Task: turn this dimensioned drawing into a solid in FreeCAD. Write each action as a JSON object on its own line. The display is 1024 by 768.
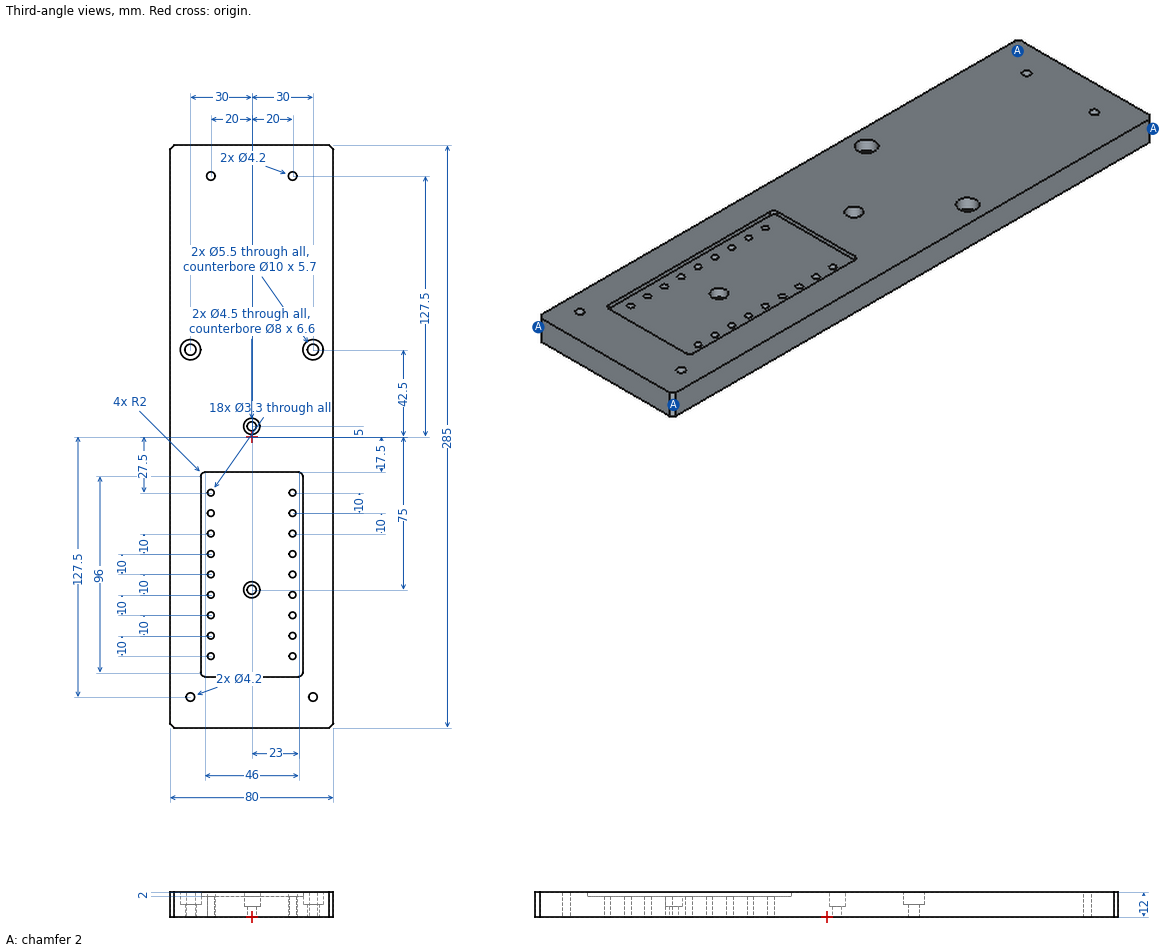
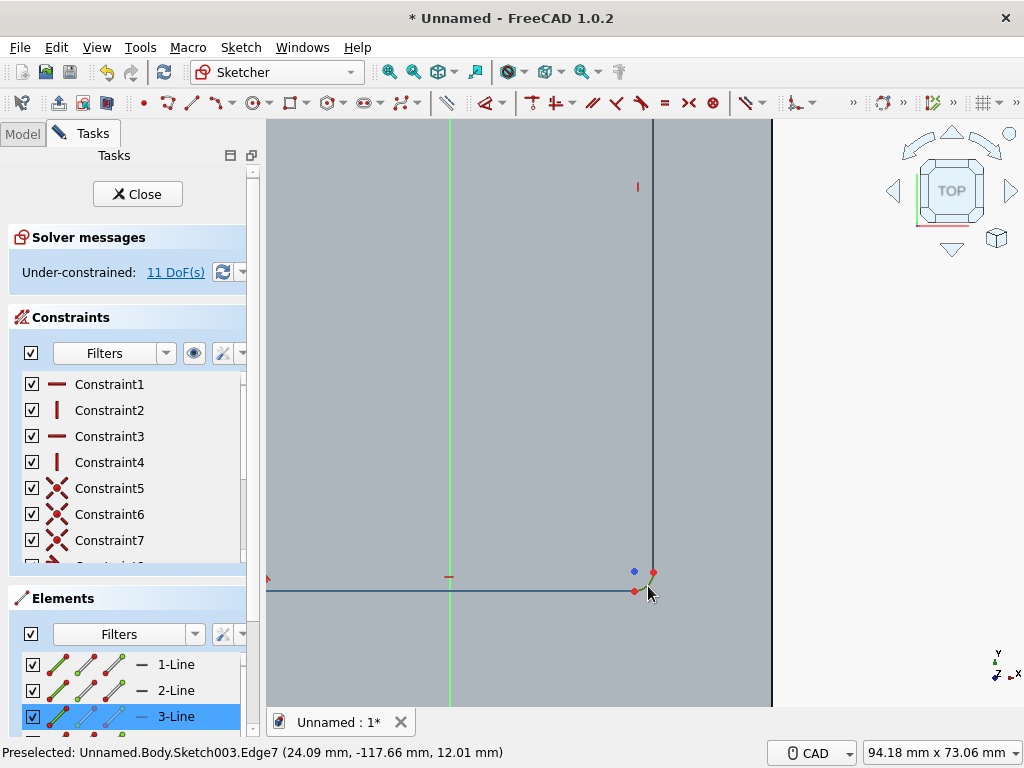
{"action": "key", "text": "t"}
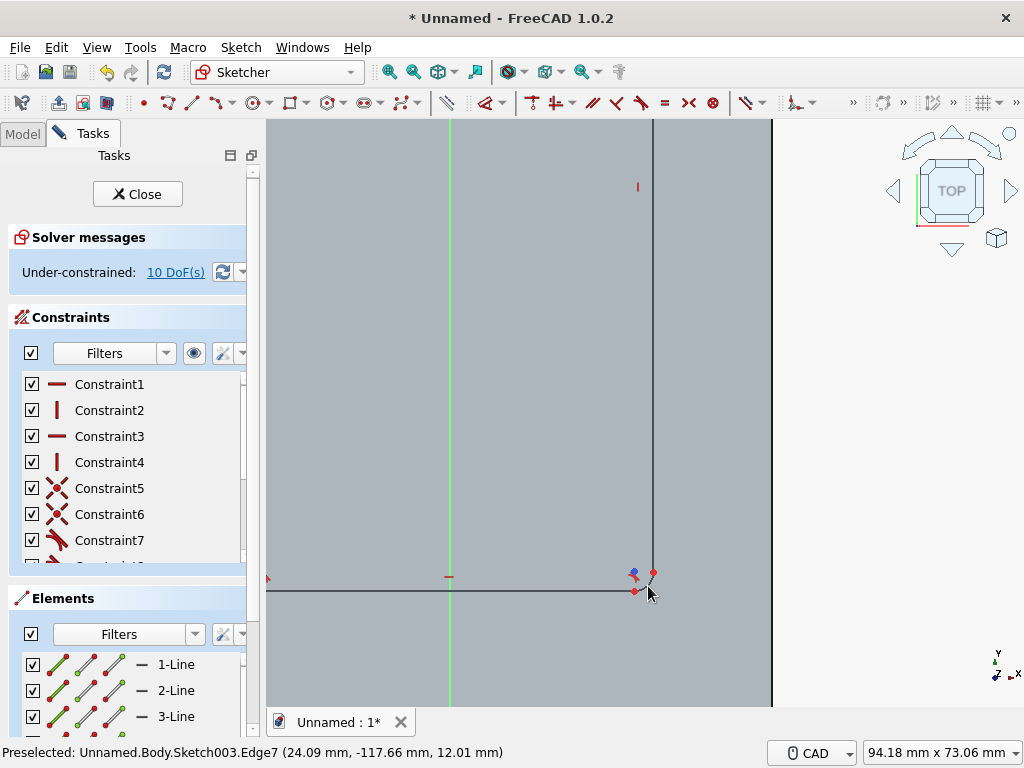
{"action": "left_click", "coordinate": [653, 341]}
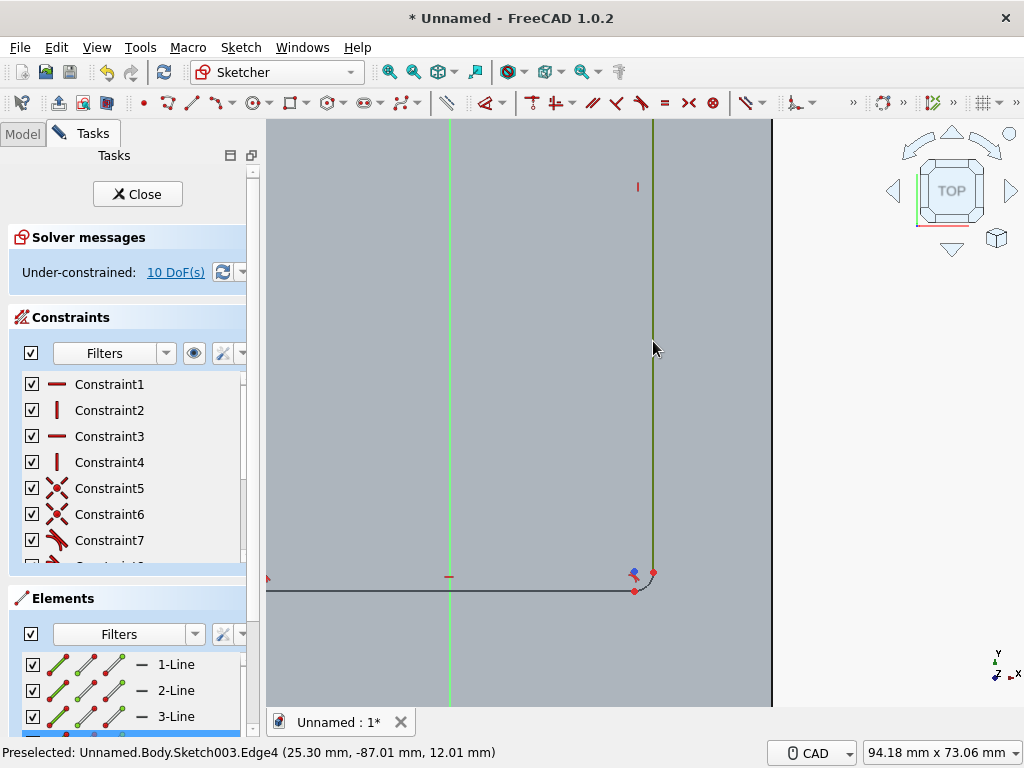
{"action": "left_click", "coordinate": [648, 586]}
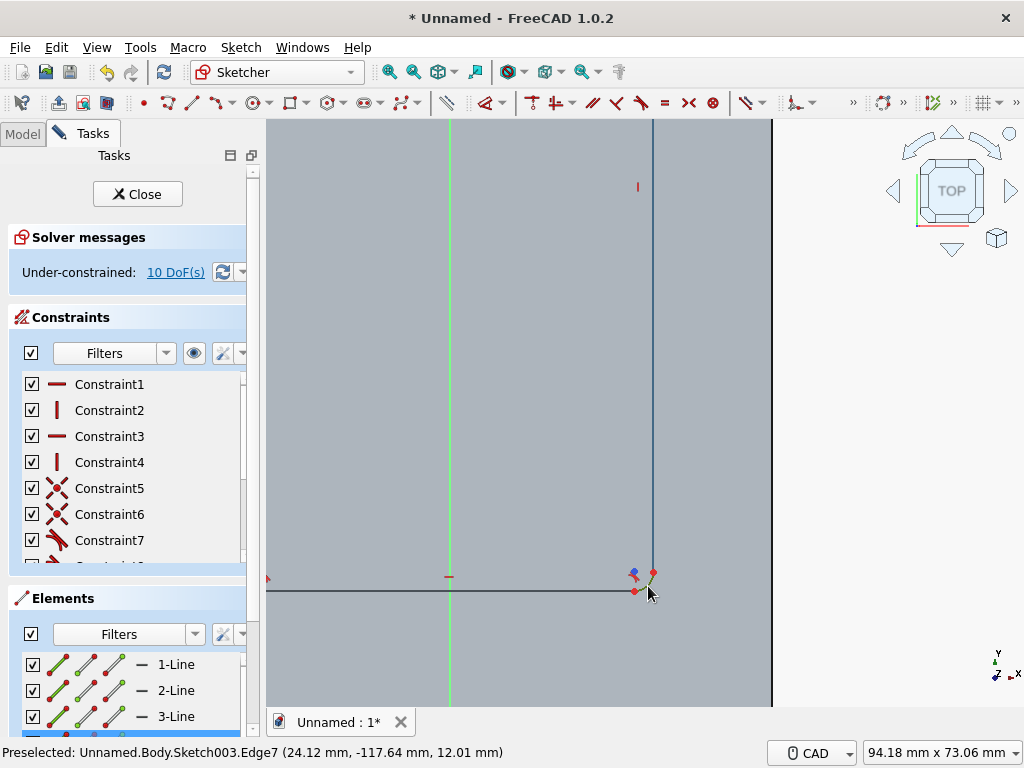
{"action": "key", "text": "t"}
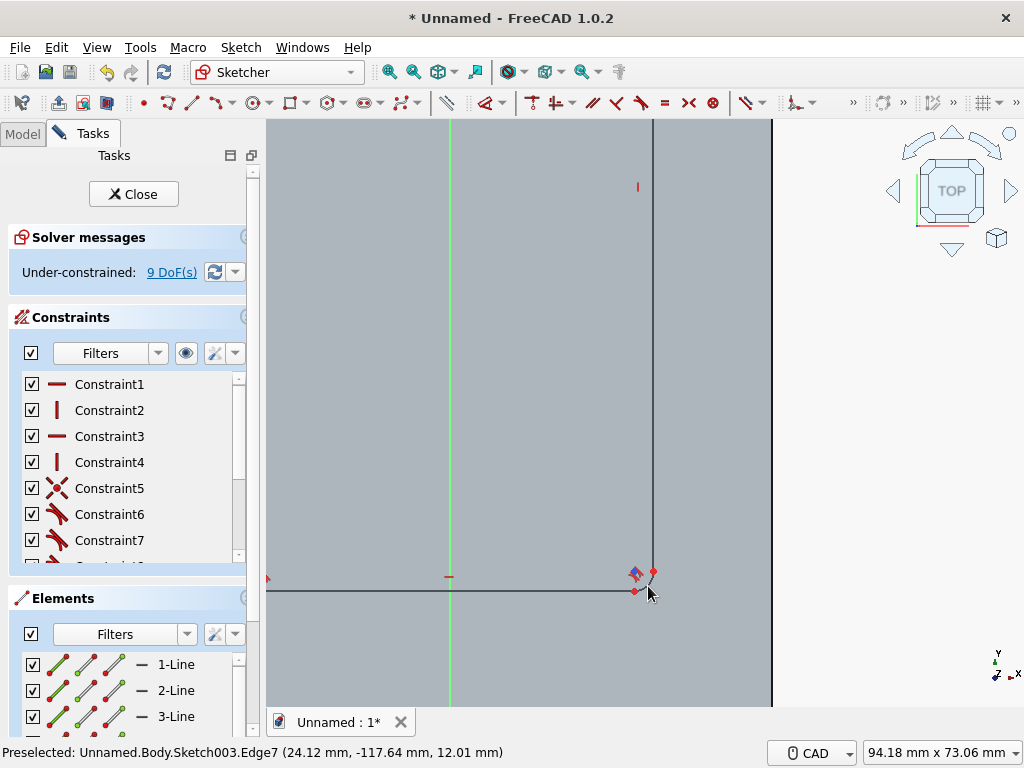
{"action": "left_click", "coordinate": [653, 341]}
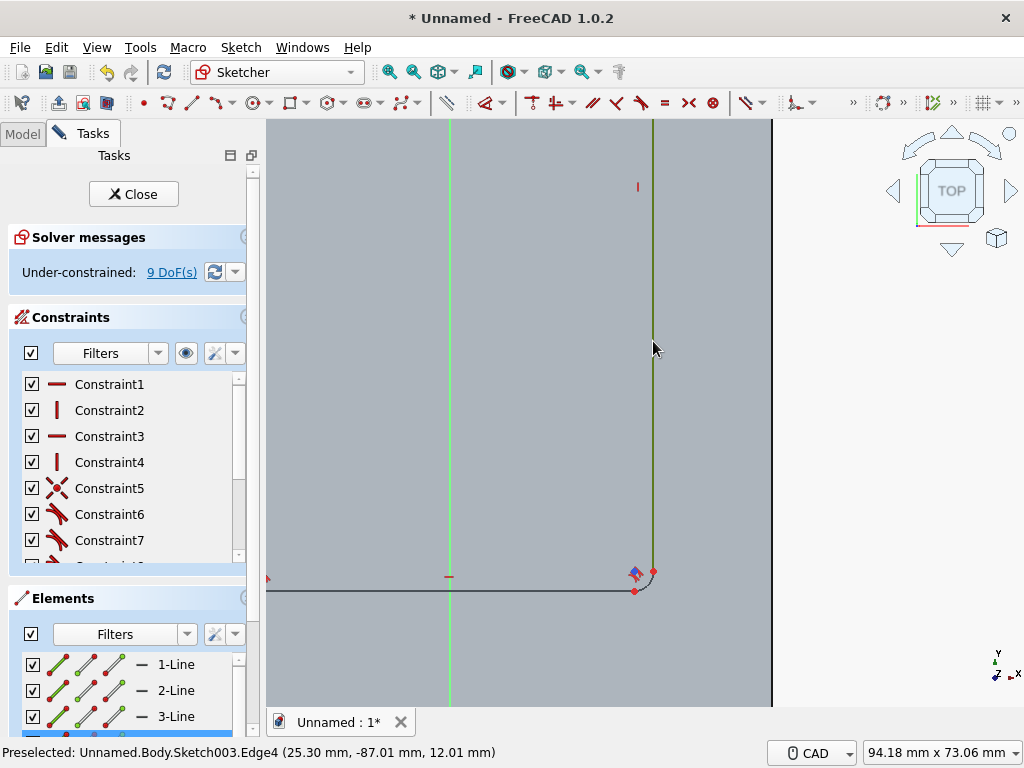
{"action": "scroll", "coordinate": [650, 587], "scroll_direction": "down", "scroll_amount": 5}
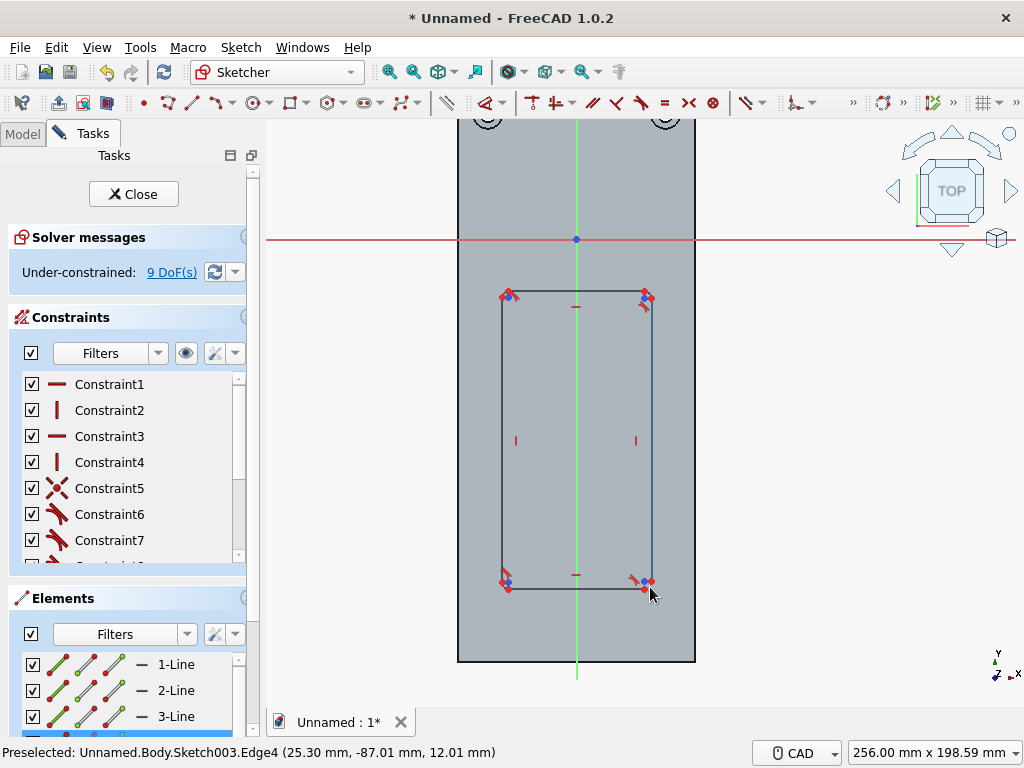
{"action": "scroll", "coordinate": [649, 293], "scroll_direction": "up", "scroll_amount": 5}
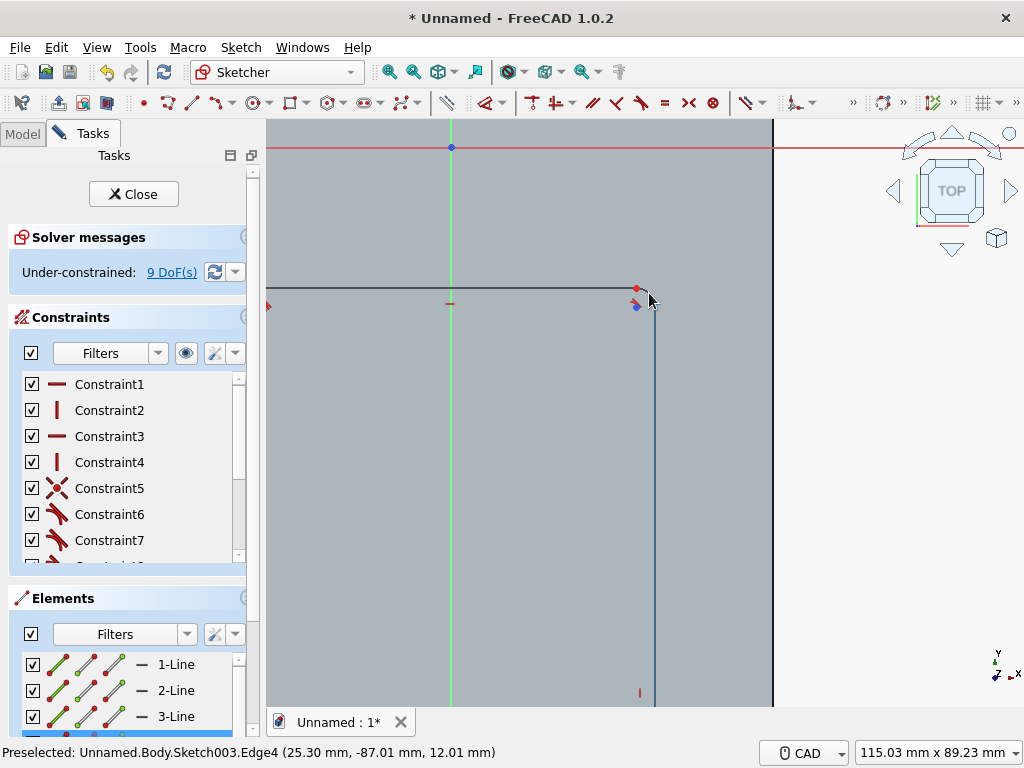
{"action": "left_click", "coordinate": [649, 294]}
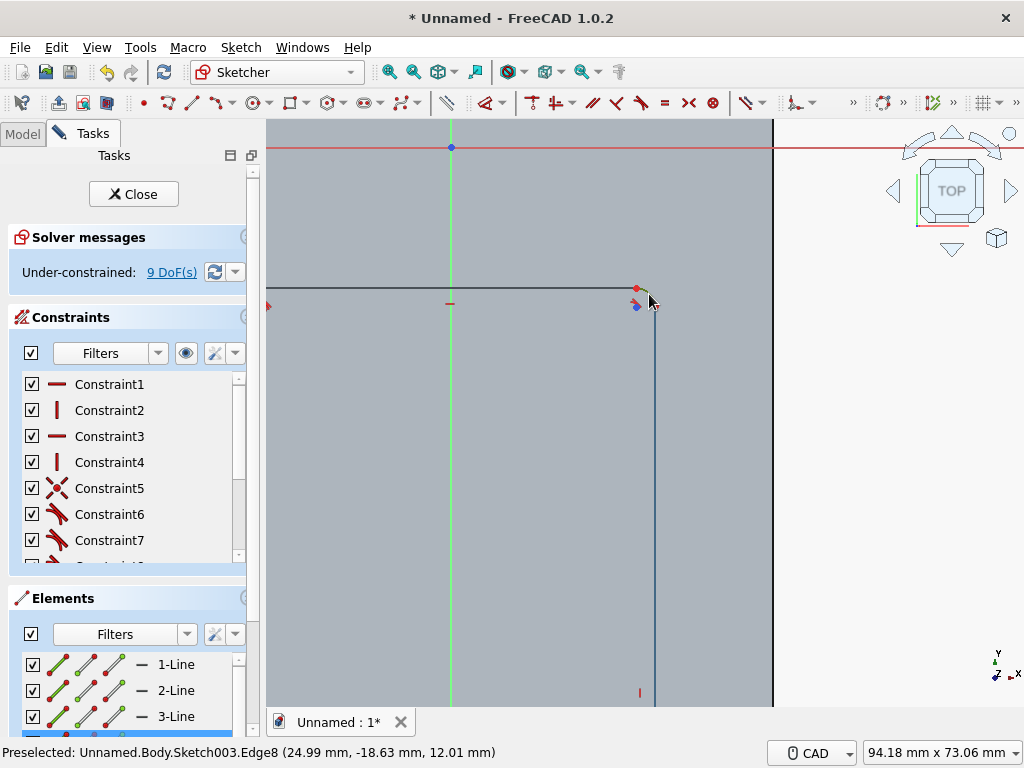
{"action": "key", "text": "t"}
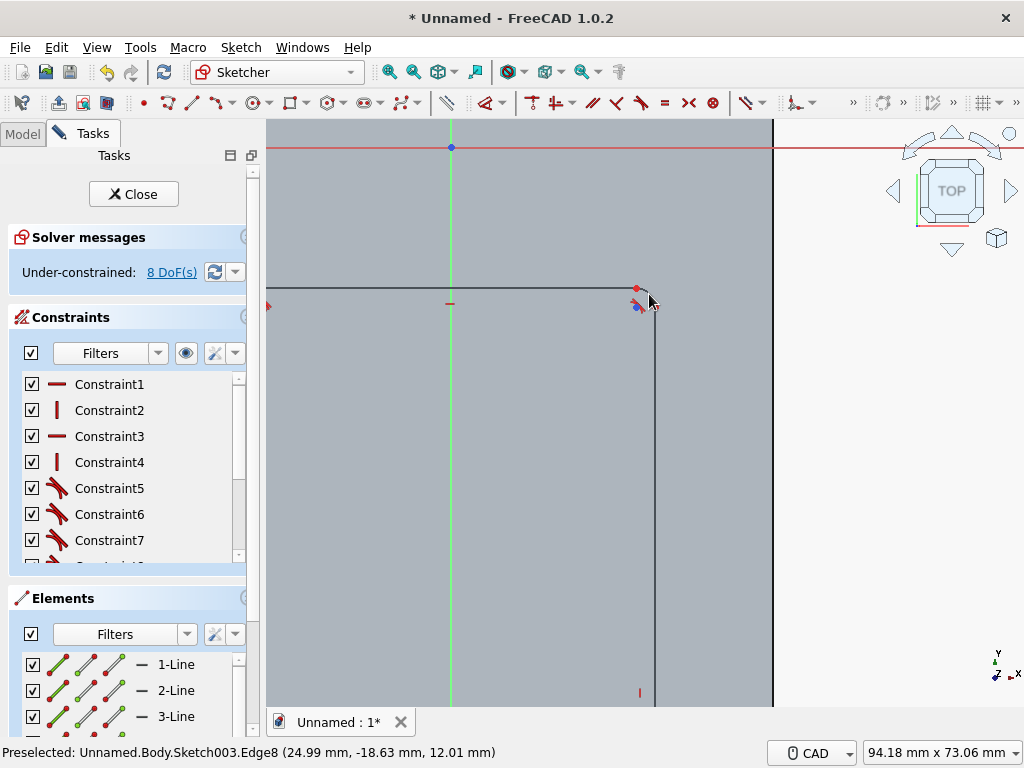
{"action": "scroll", "coordinate": [649, 292], "scroll_direction": "down", "scroll_amount": 5}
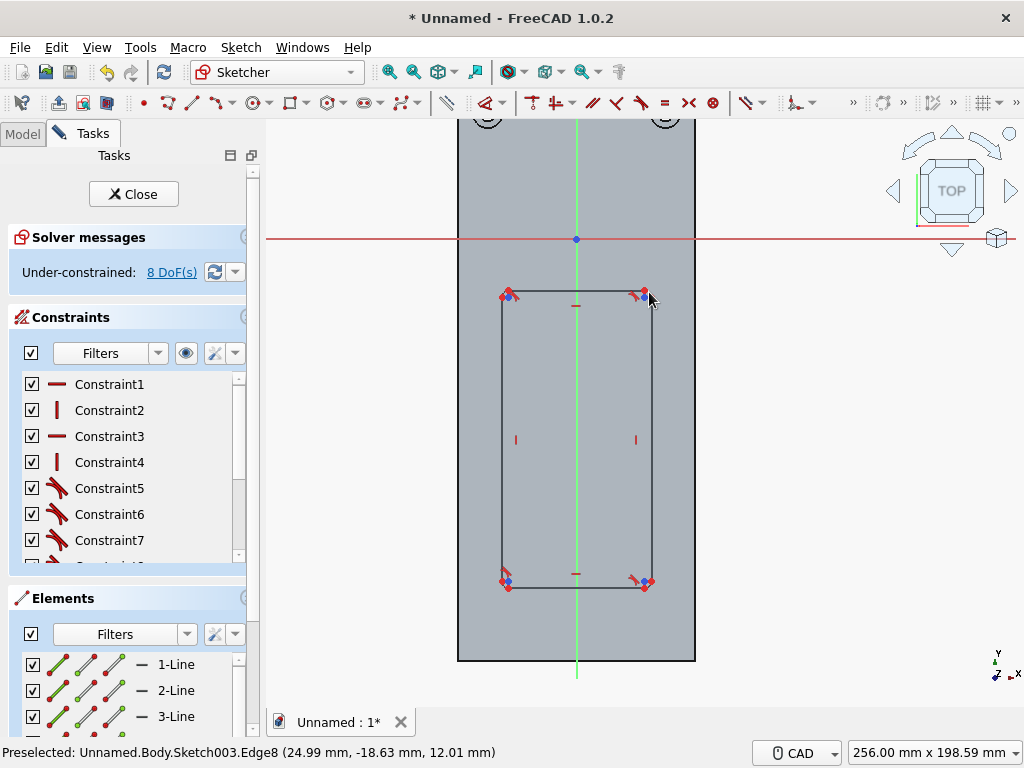
{"action": "scroll", "coordinate": [504, 293], "scroll_direction": "up", "scroll_amount": 6}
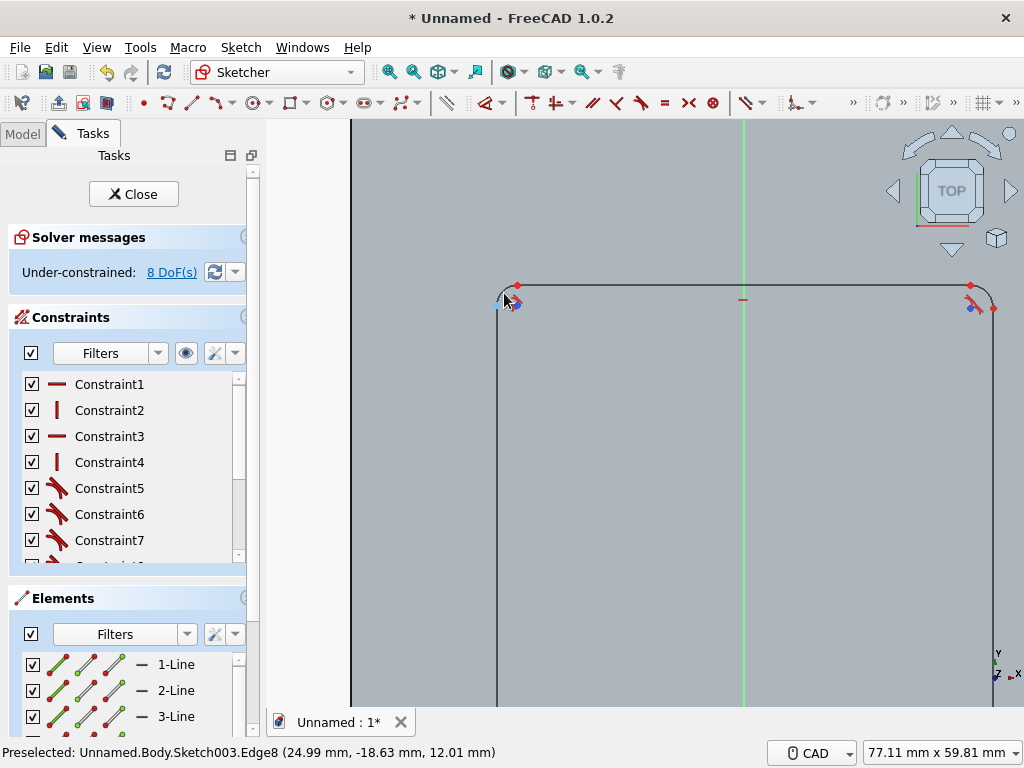
{"action": "left_click", "coordinate": [503, 291]}